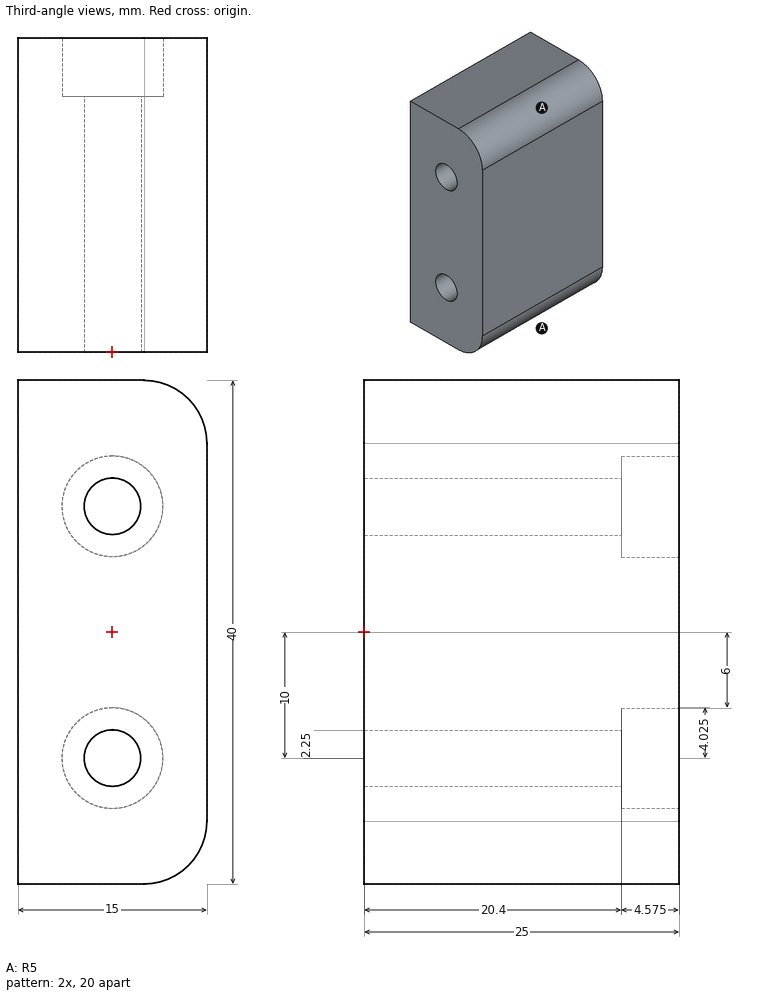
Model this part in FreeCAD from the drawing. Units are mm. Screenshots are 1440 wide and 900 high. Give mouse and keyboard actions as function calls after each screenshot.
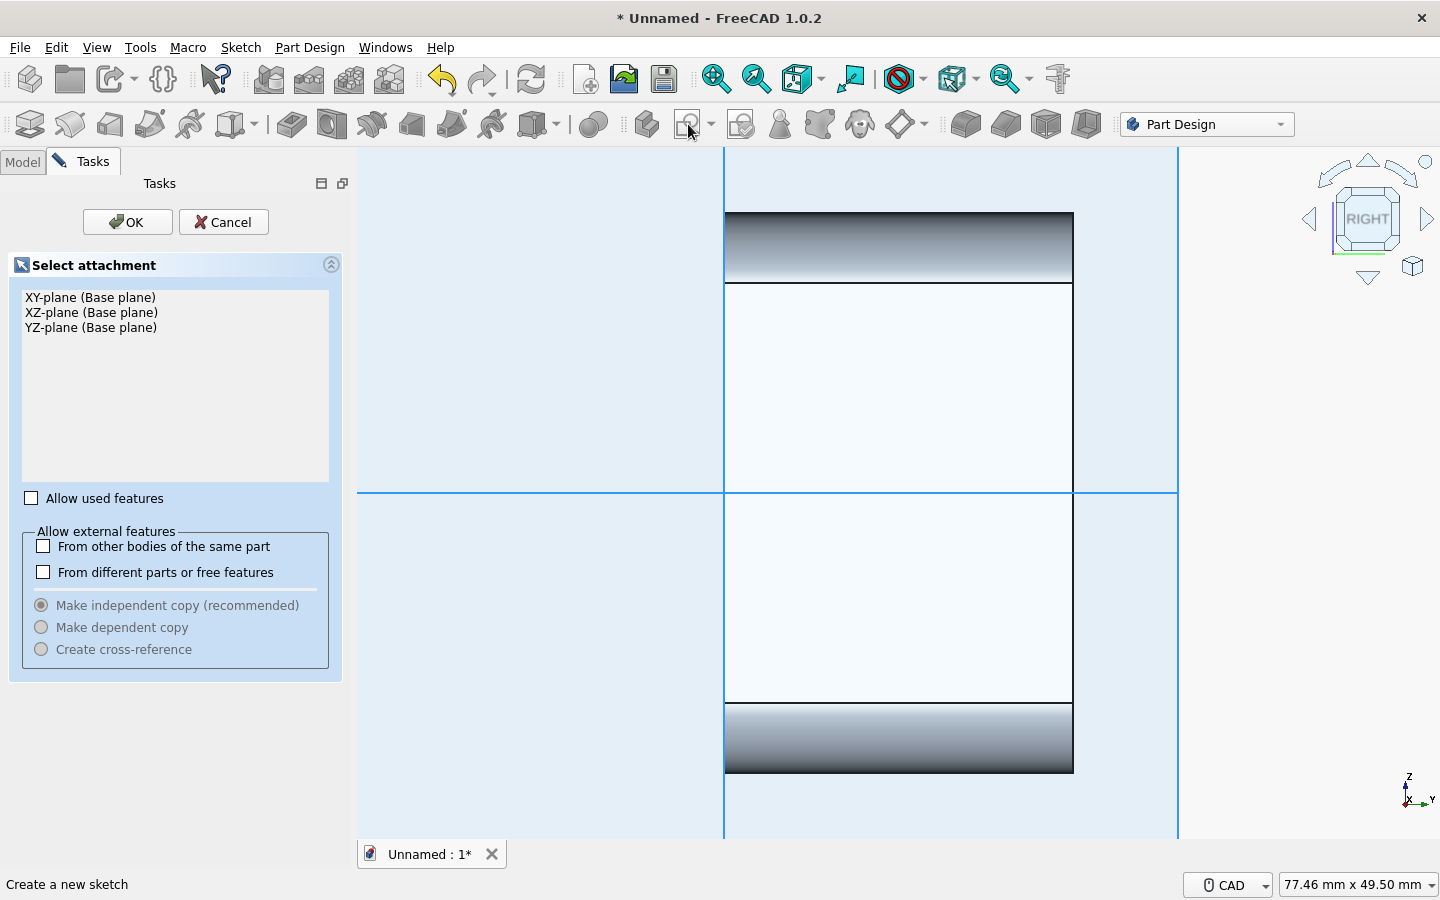
click(82, 328)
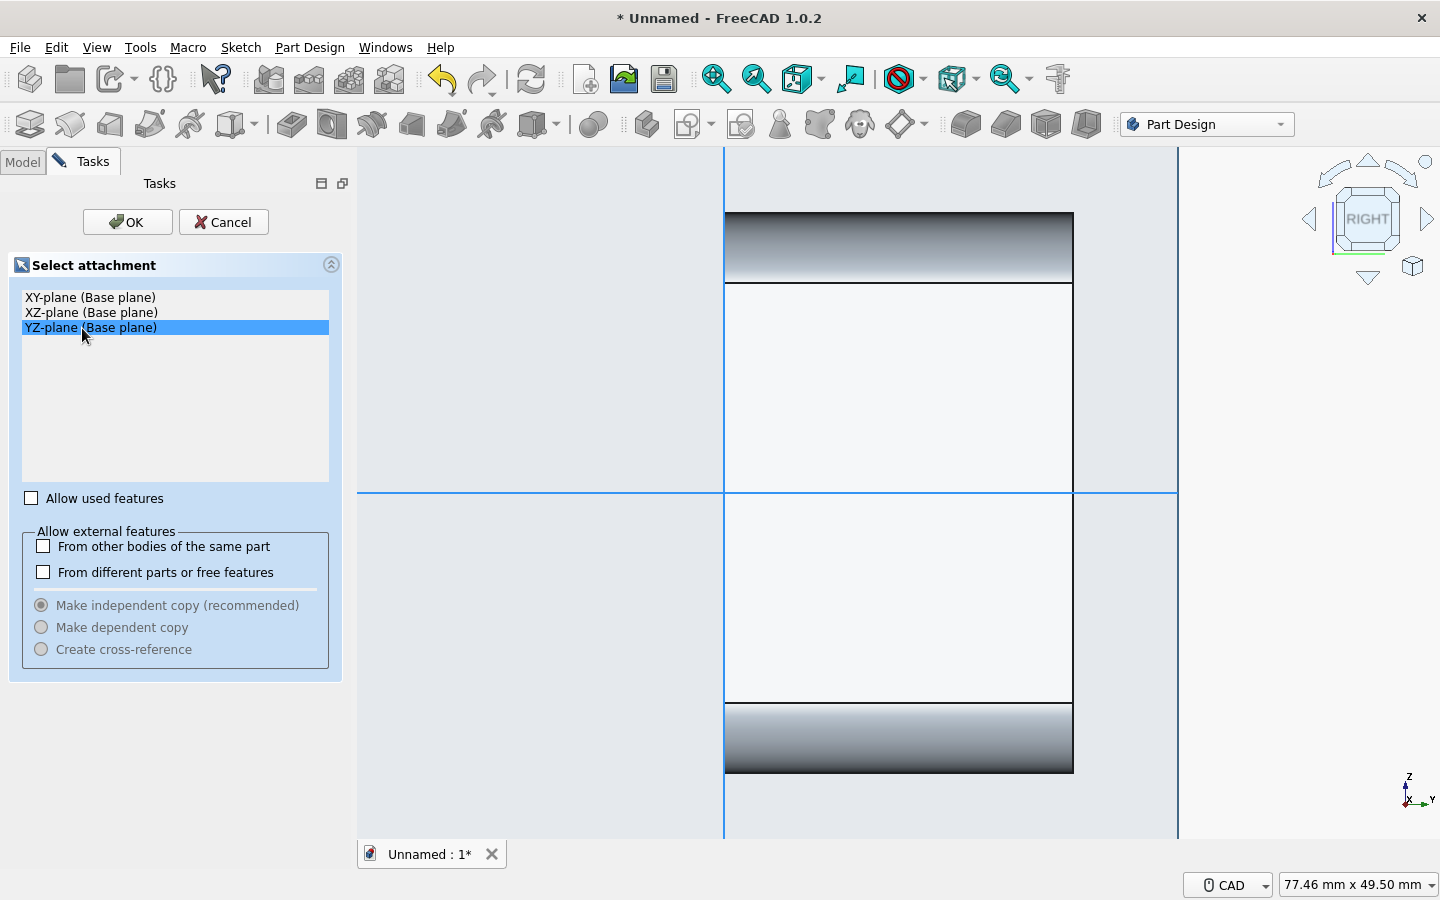
click(128, 222)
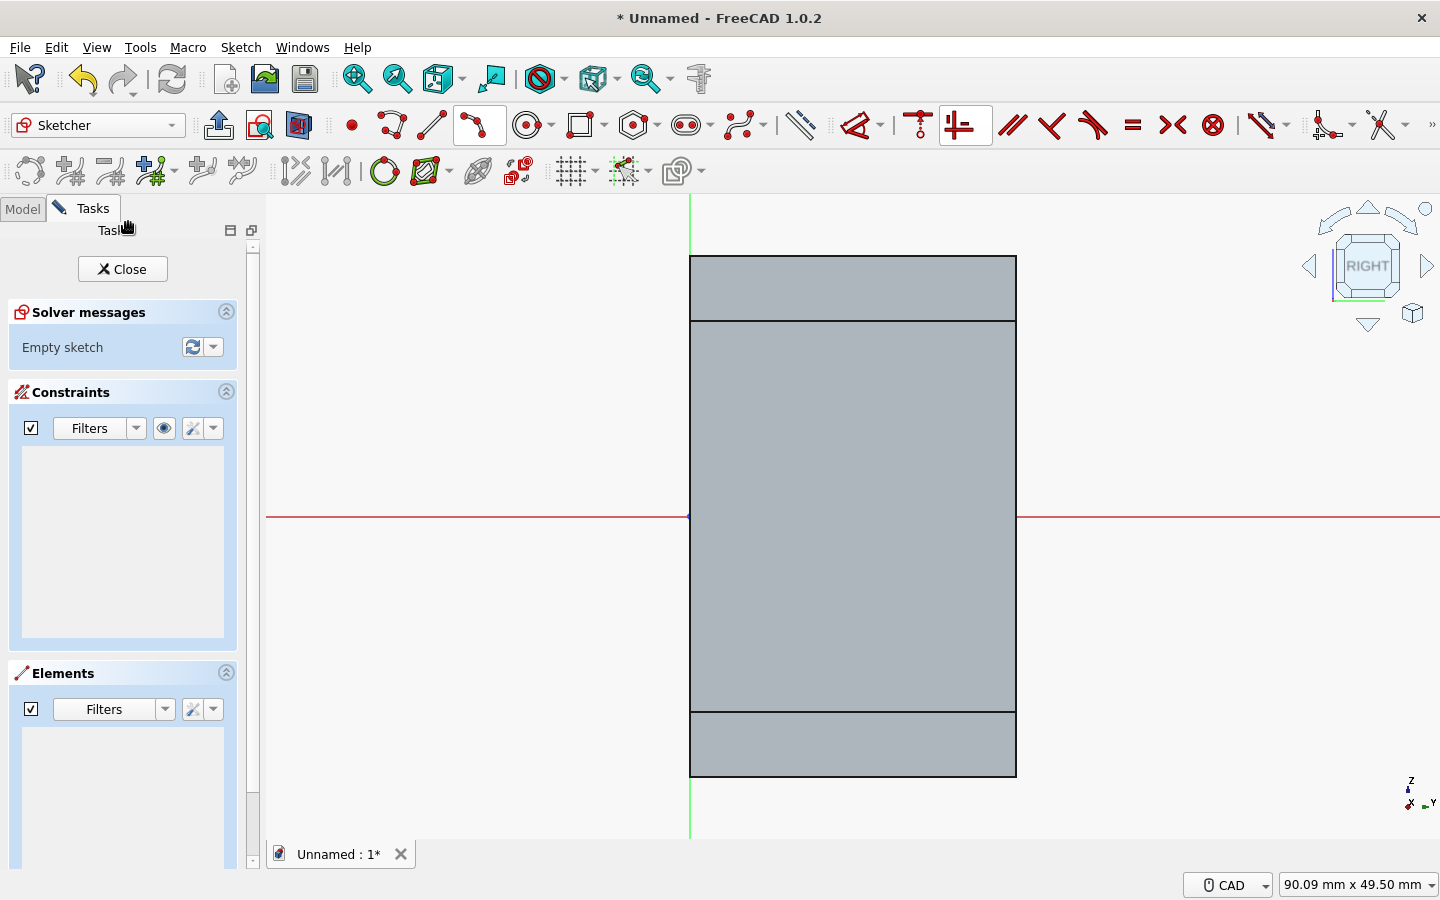
click(300, 126)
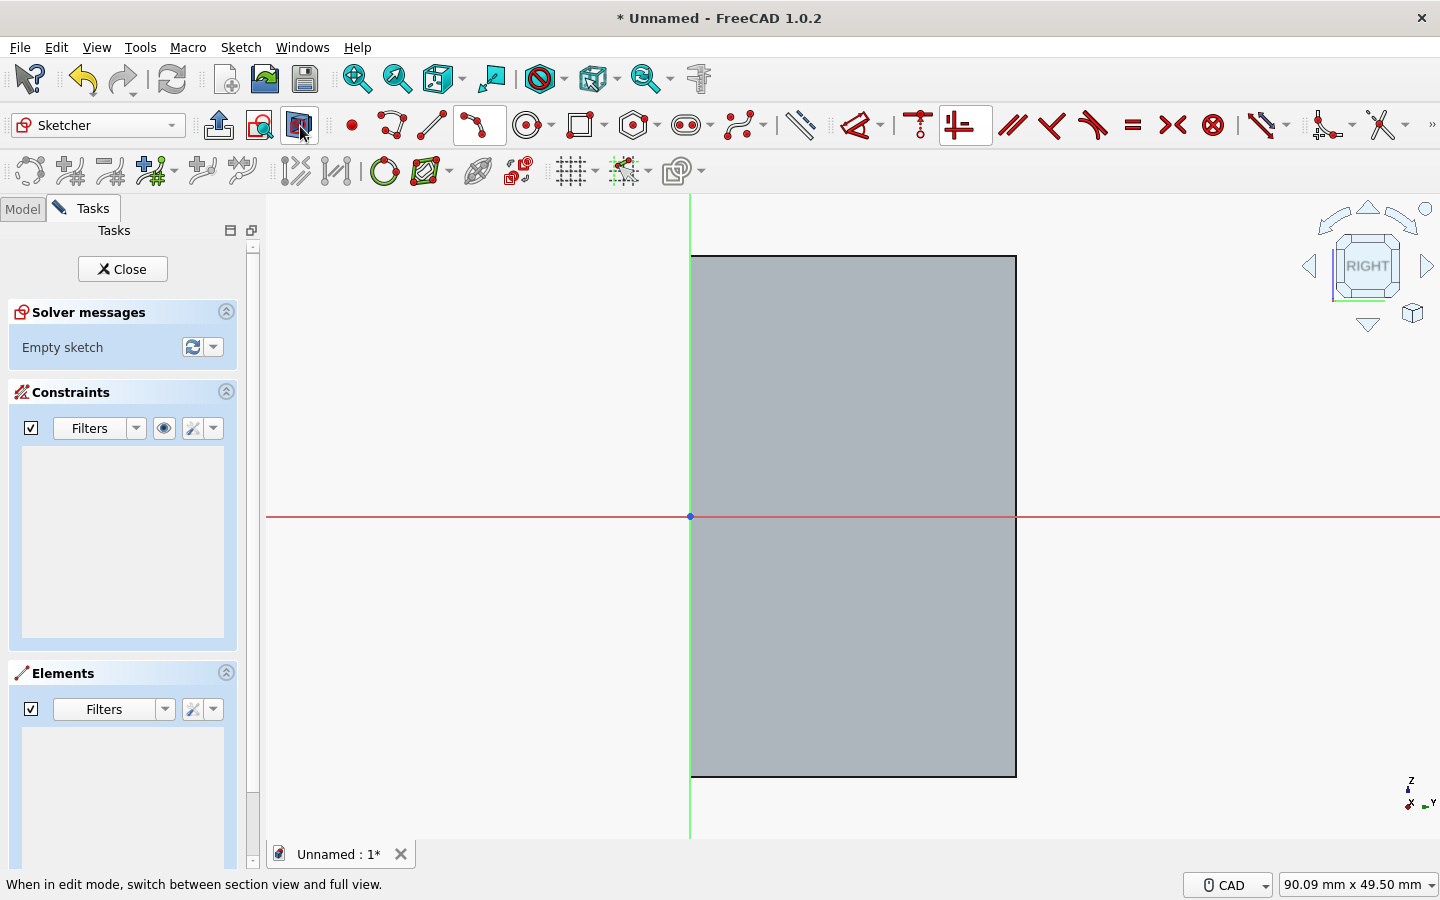
scroll(795, 714, up, 2)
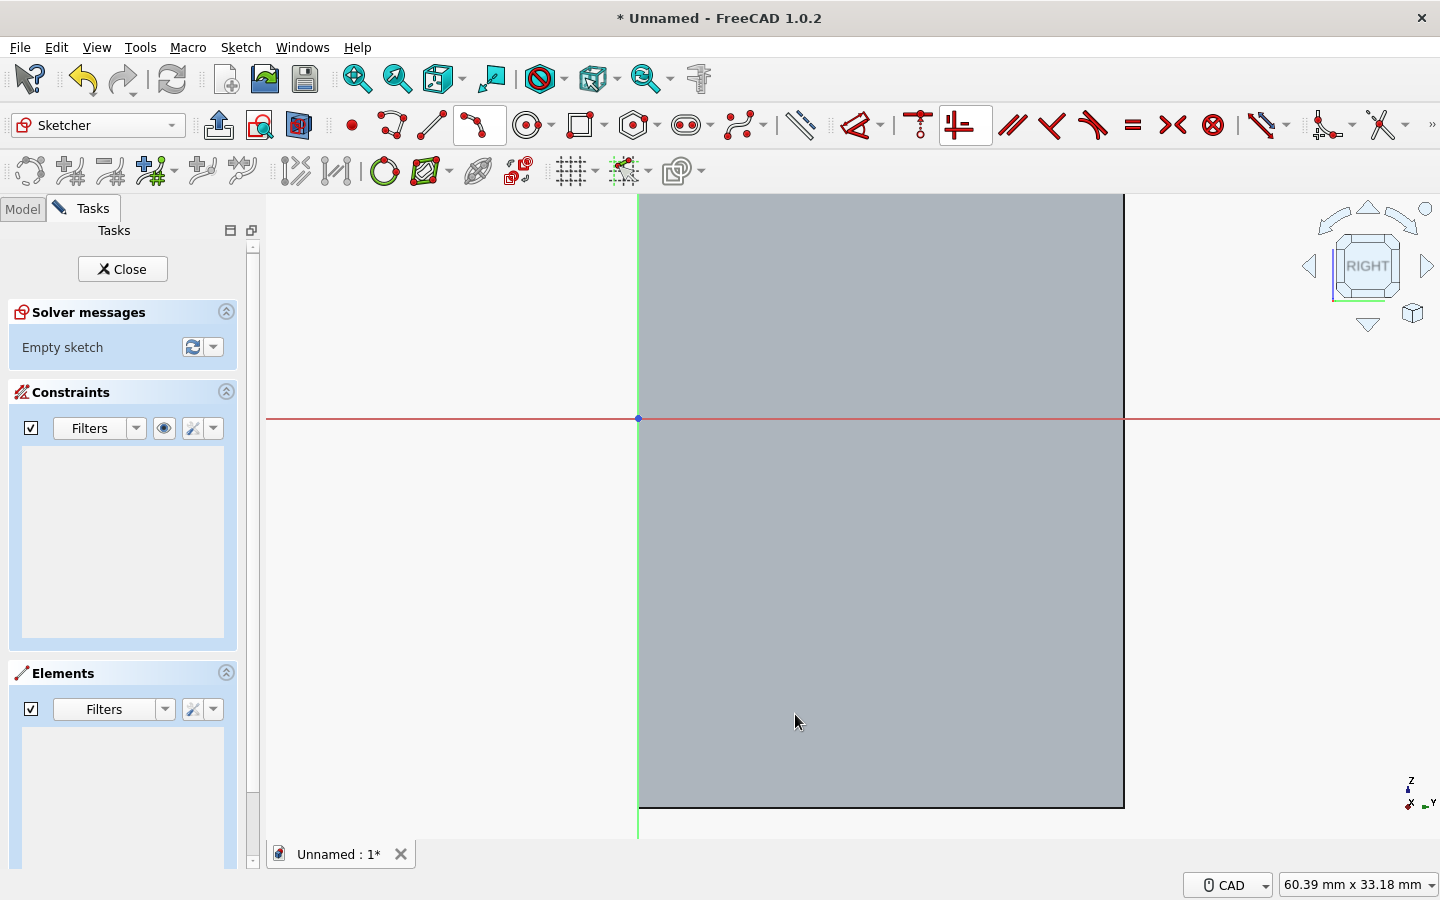
click(392, 126)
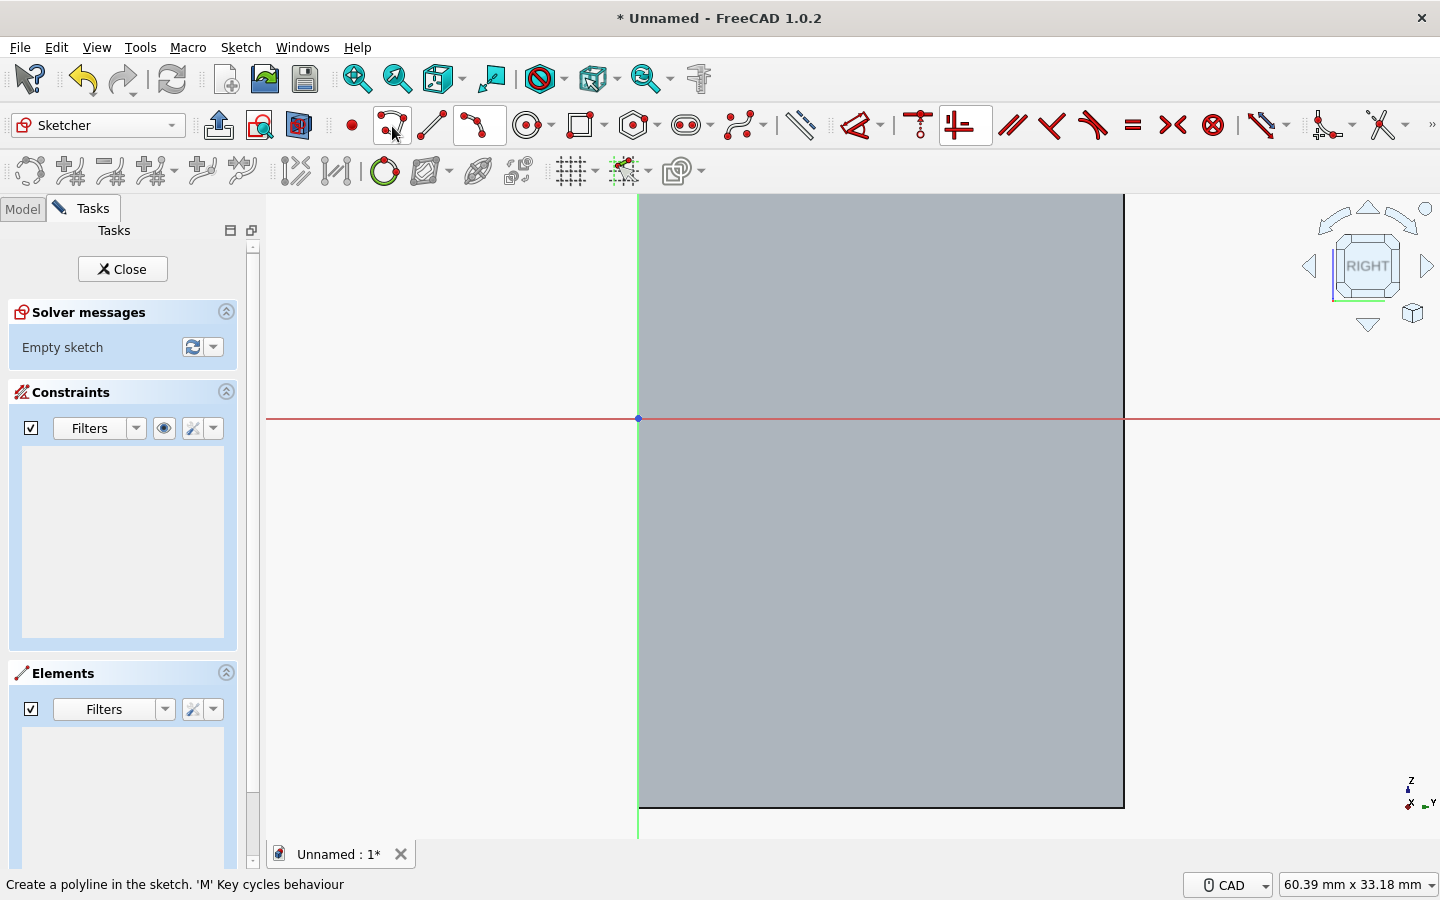
click(638, 570)
click(647, 613)
click(1124, 613)
click(1124, 535)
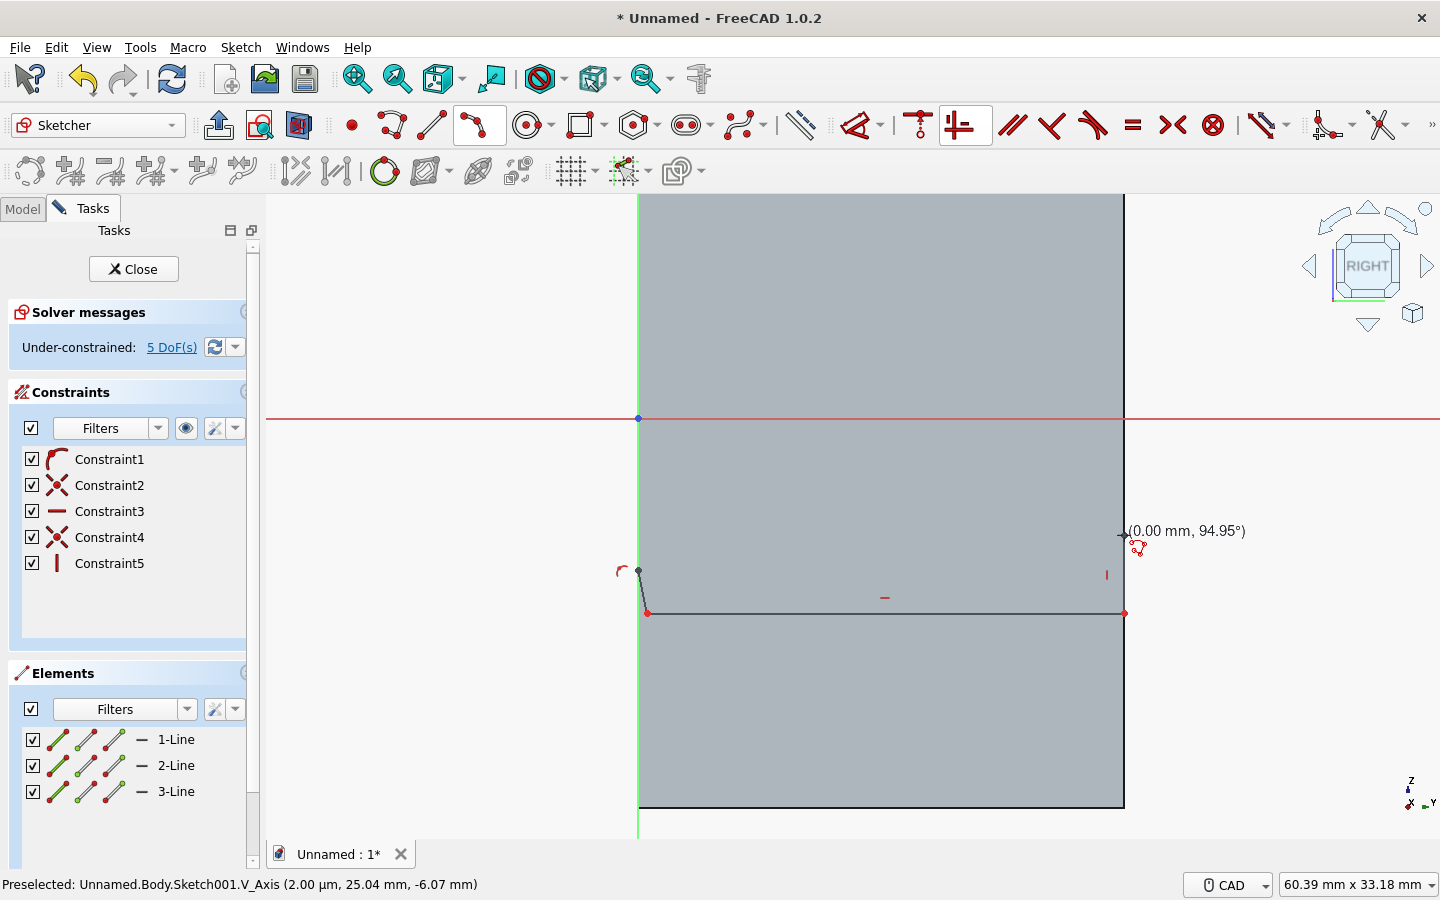
scroll(1124, 536, up, 18)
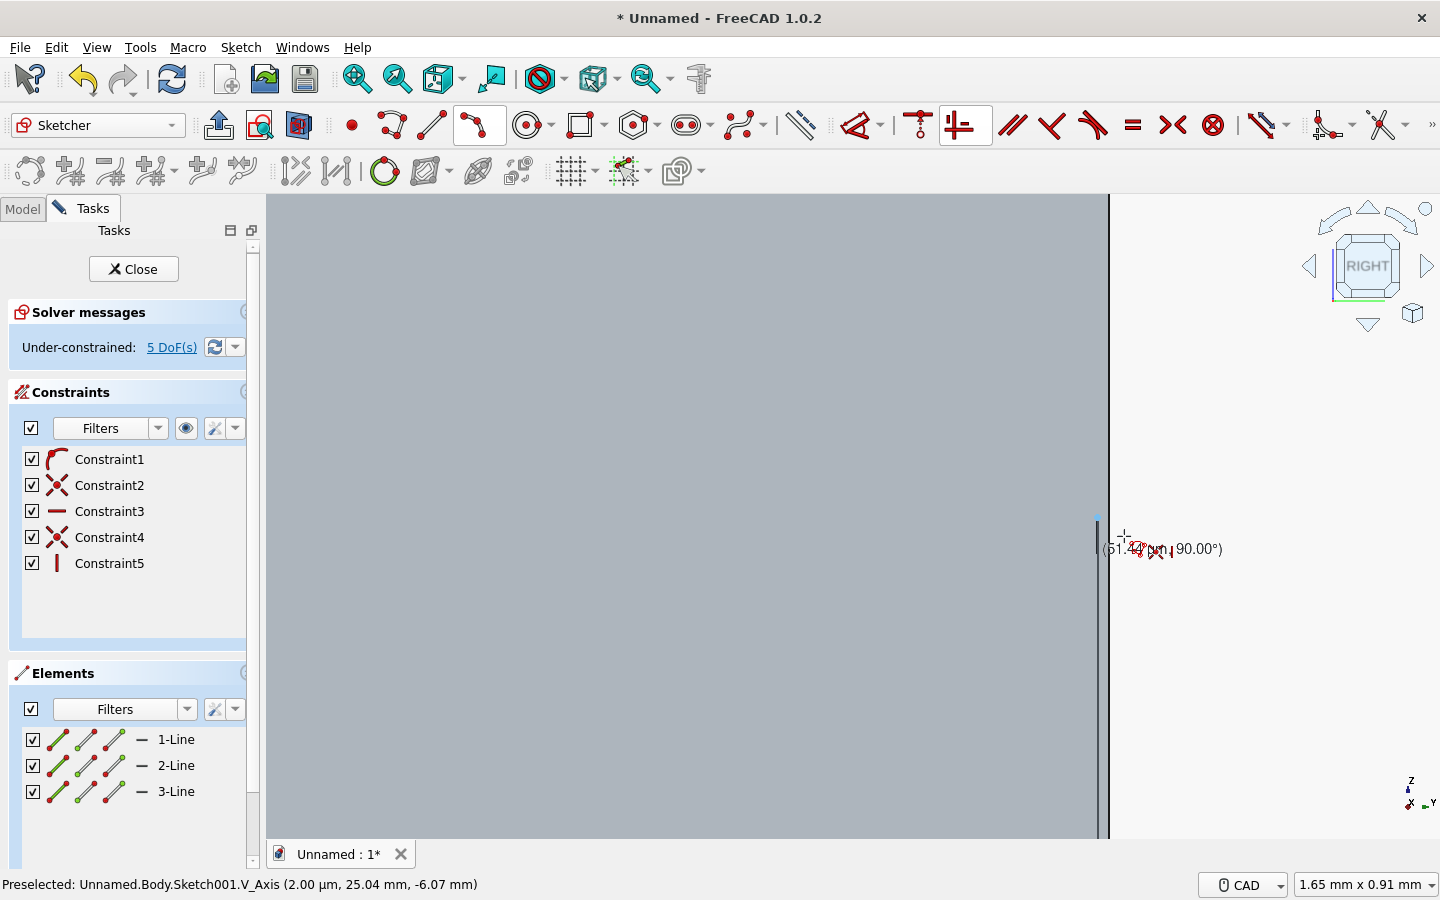
click(1091, 503)